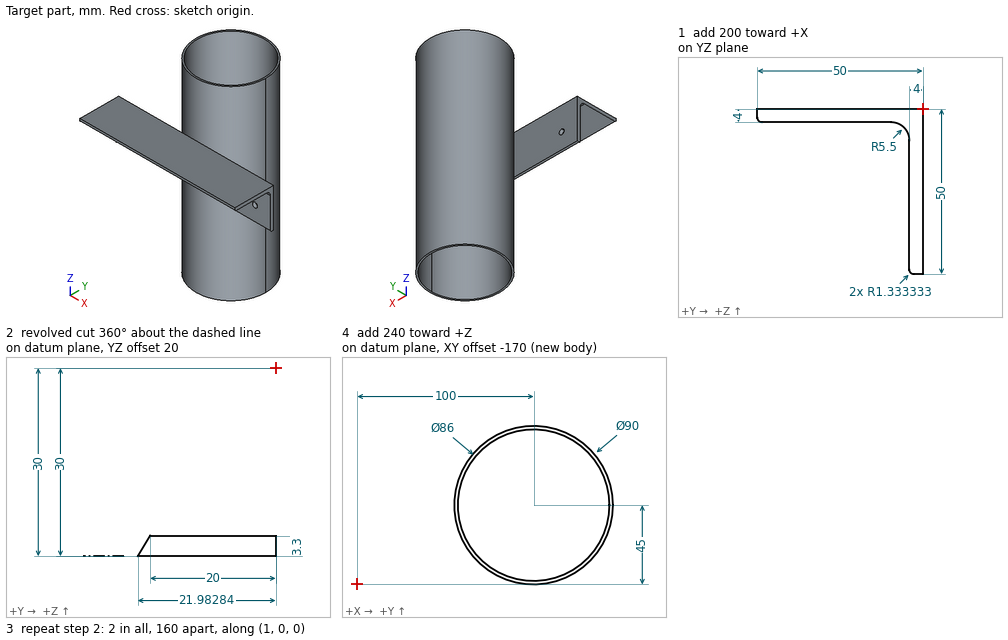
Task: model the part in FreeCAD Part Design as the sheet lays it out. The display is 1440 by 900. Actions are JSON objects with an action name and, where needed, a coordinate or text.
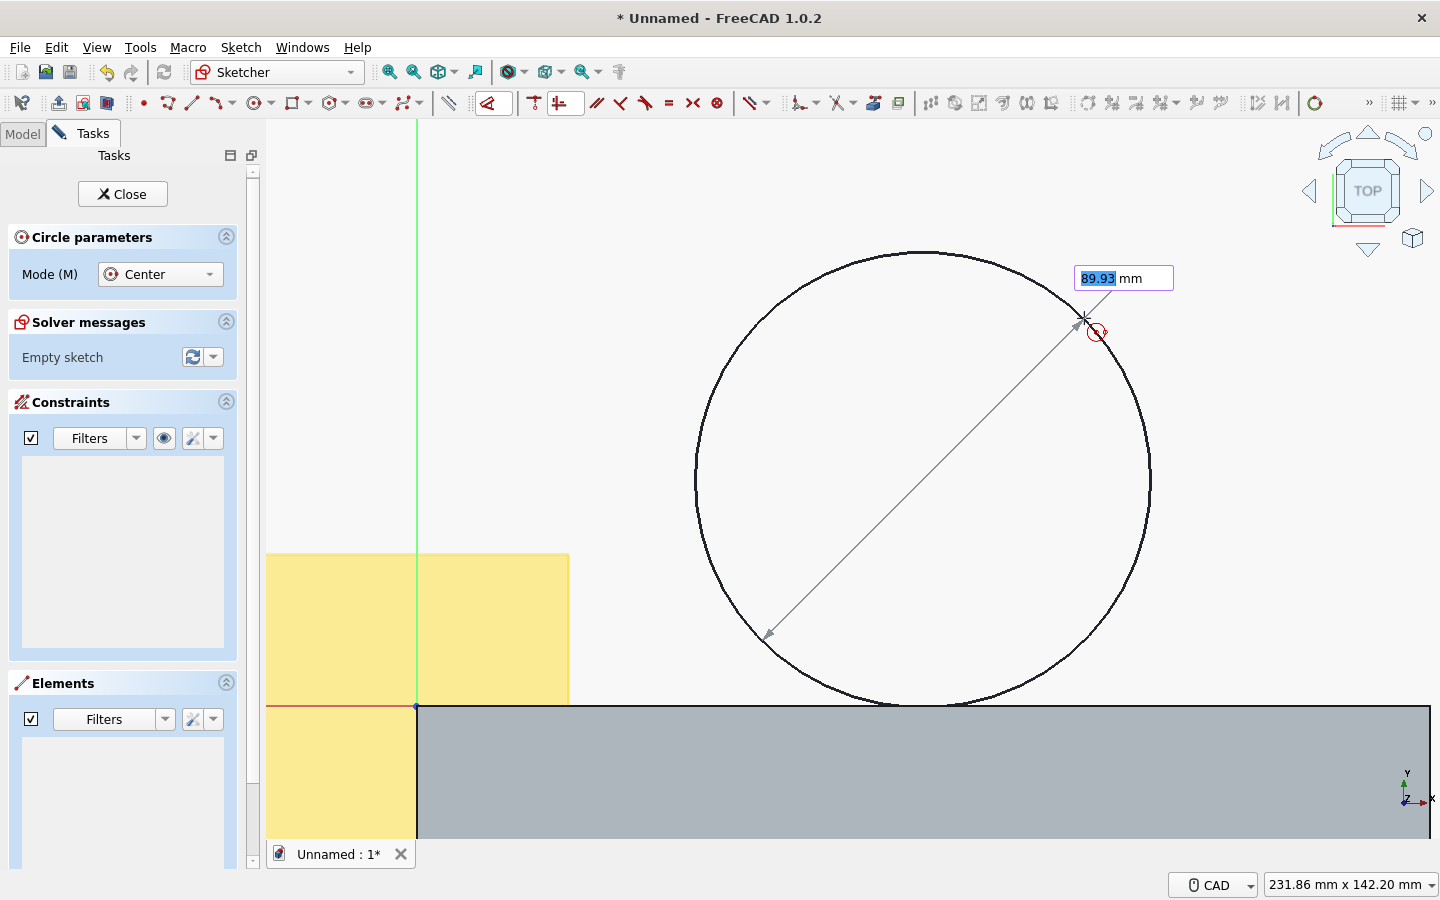
{"action": "type", "text": "90"}
{"action": "key", "text": "Return"}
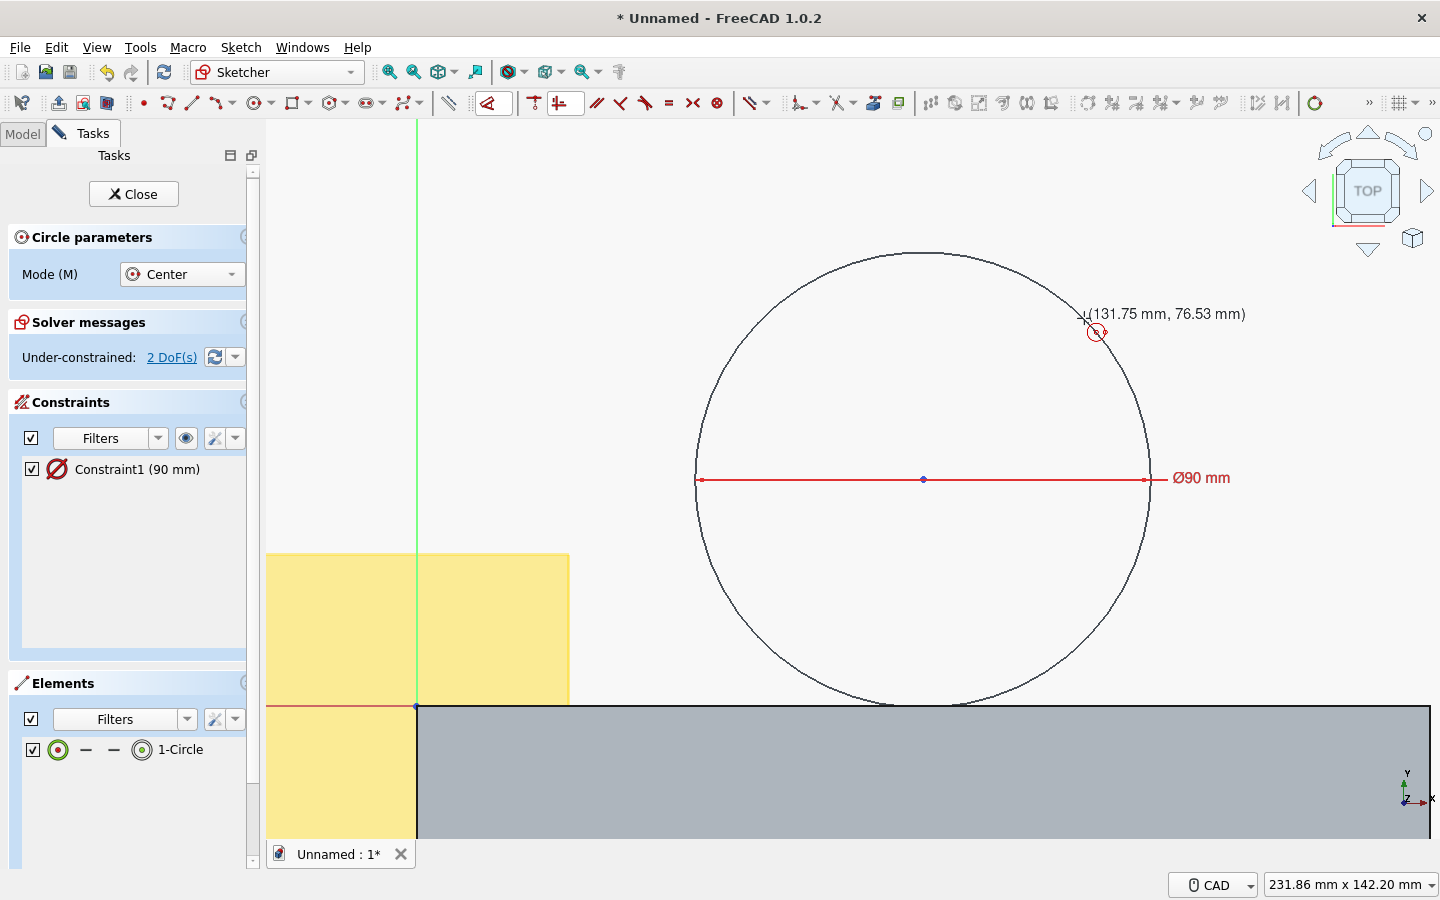
{"action": "left_click", "coordinate": [923, 480]}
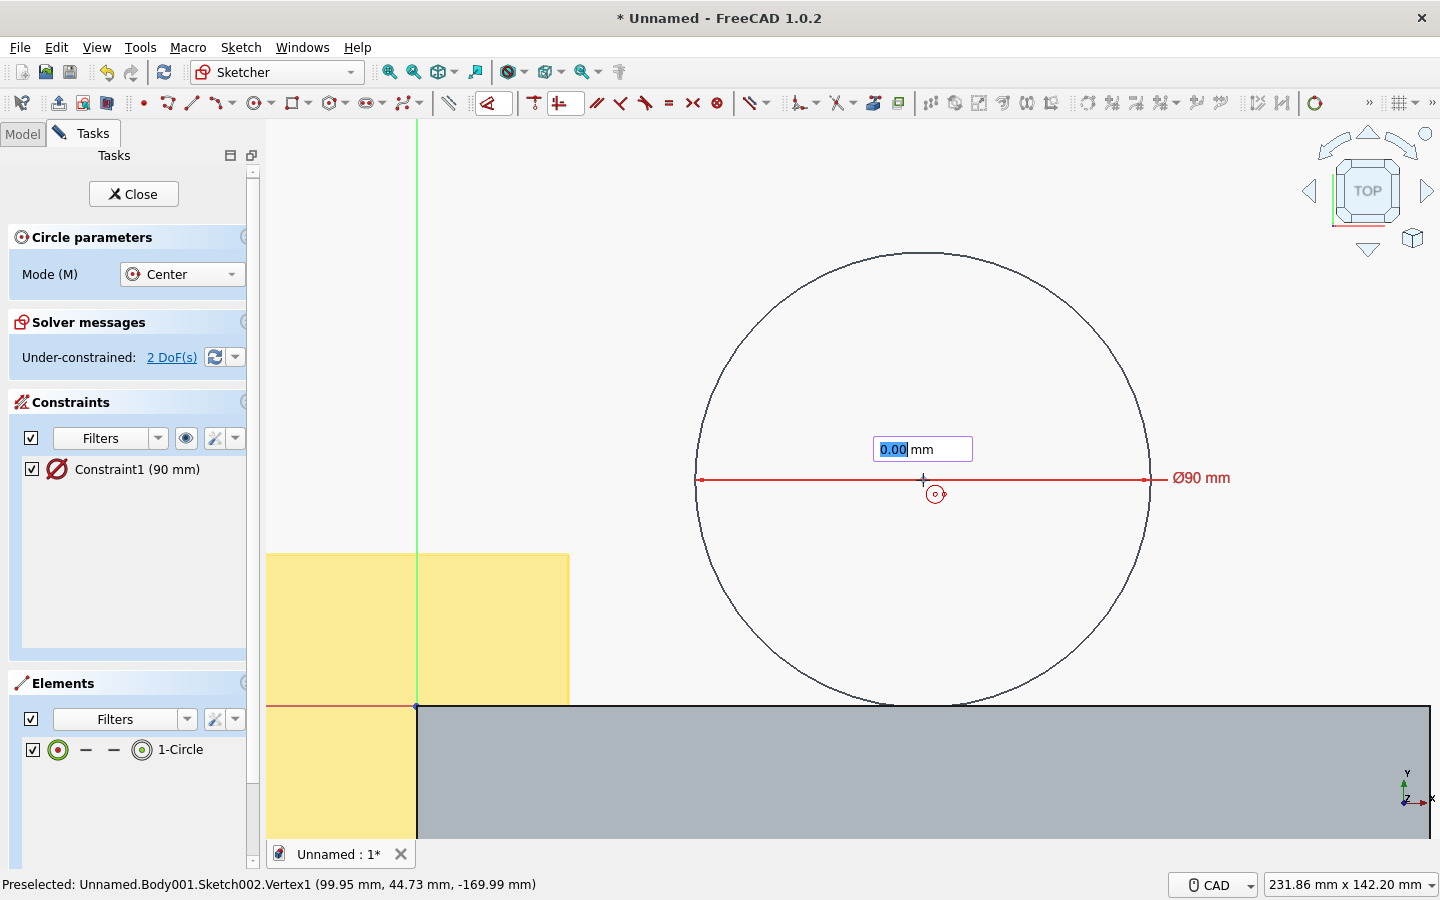
{"action": "scroll", "coordinate": [1077, 325], "scroll_direction": "up", "scroll_amount": 3}
{"action": "mouse_move", "coordinate": [1077, 324]}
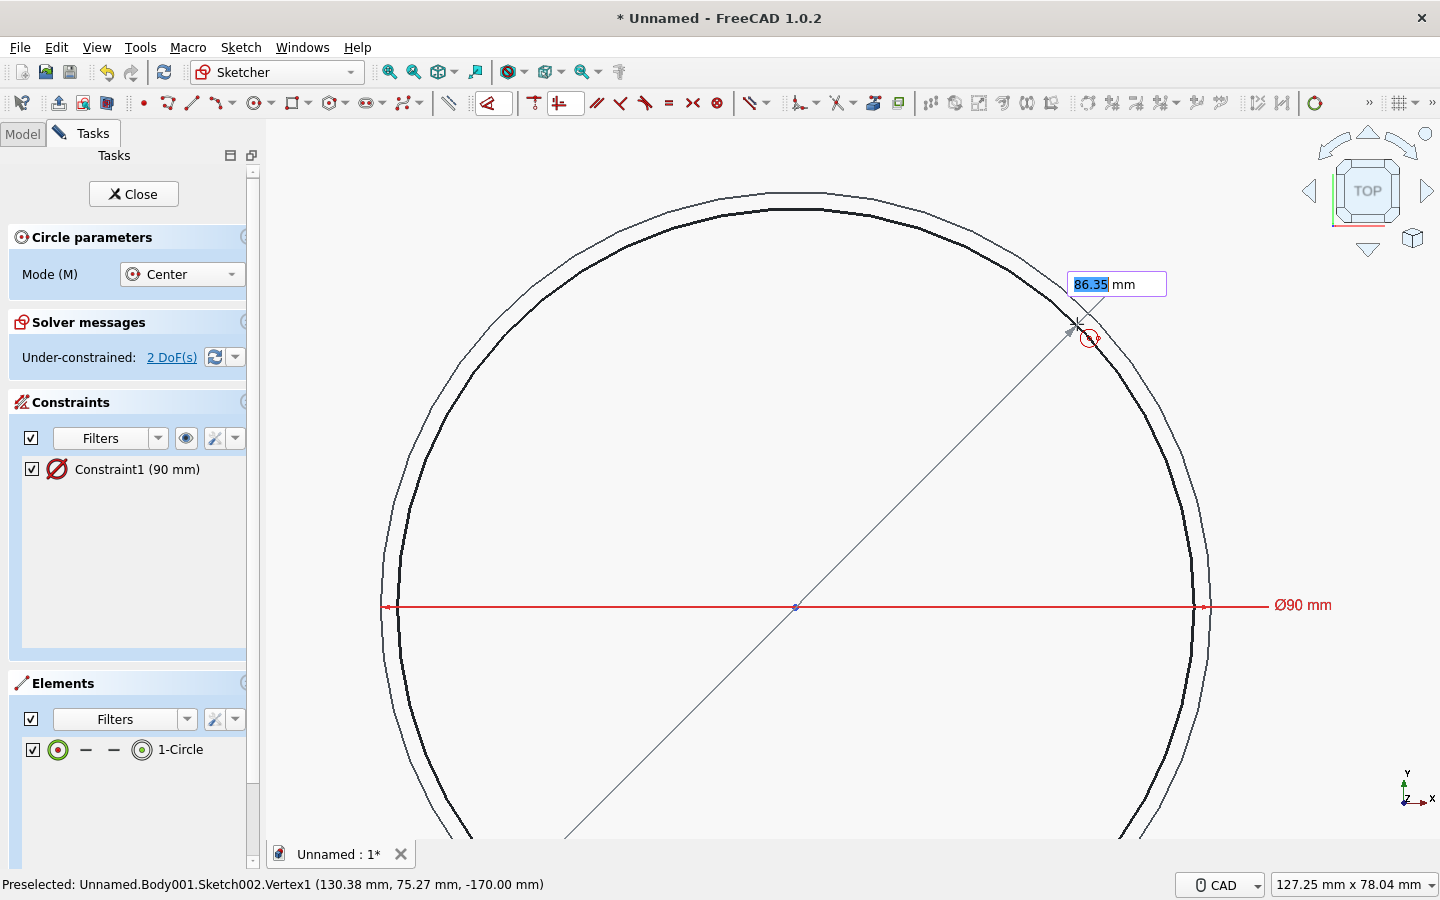
{"action": "type", "text": "86"}
{"action": "key", "text": "Return"}
{"action": "key", "text": "Escape"}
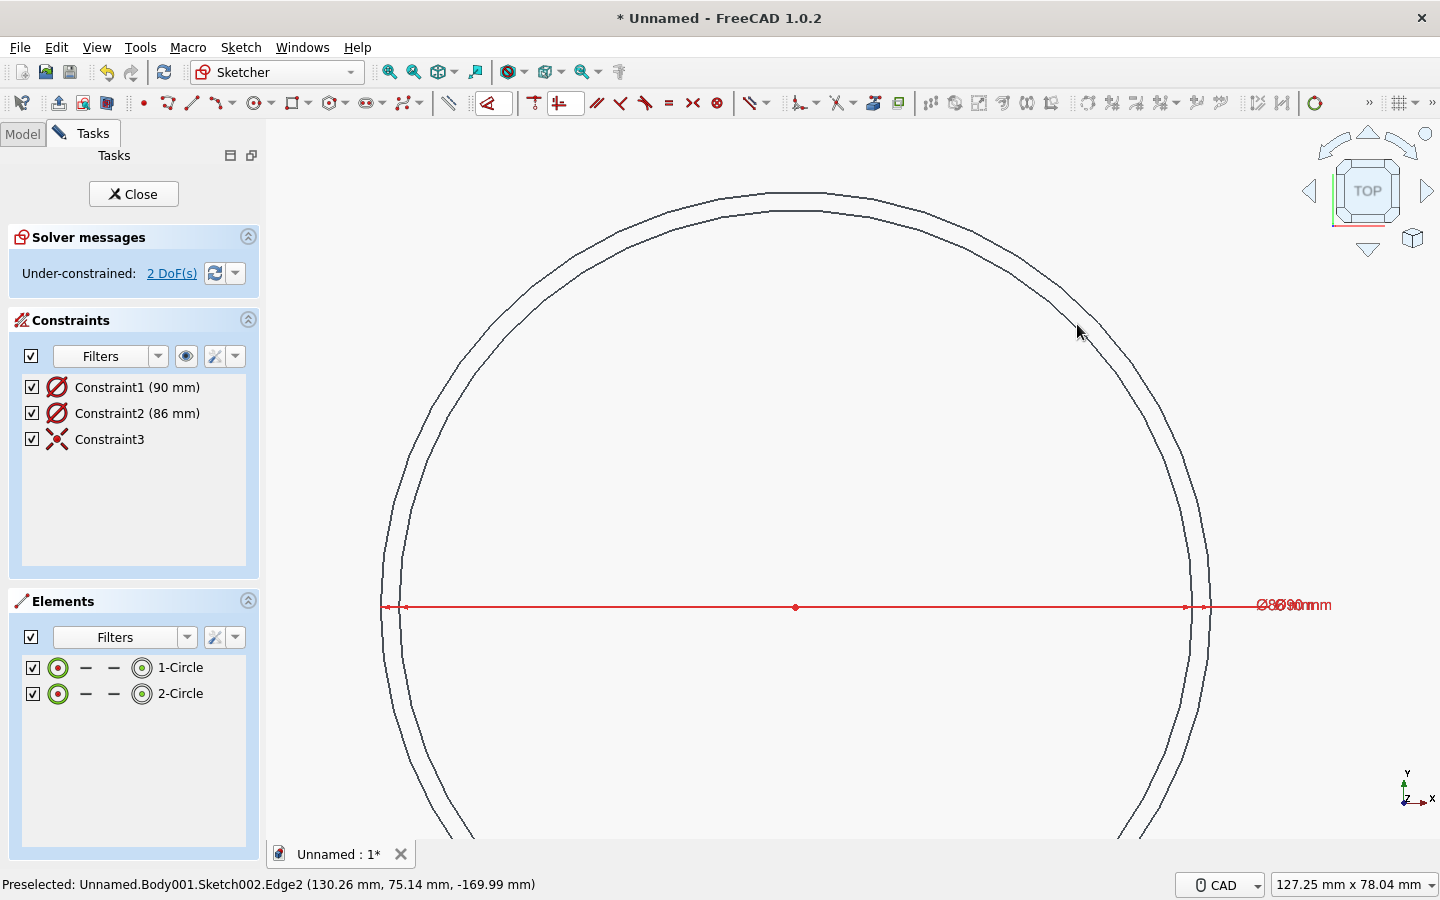
{"action": "left_click", "coordinate": [796, 607]}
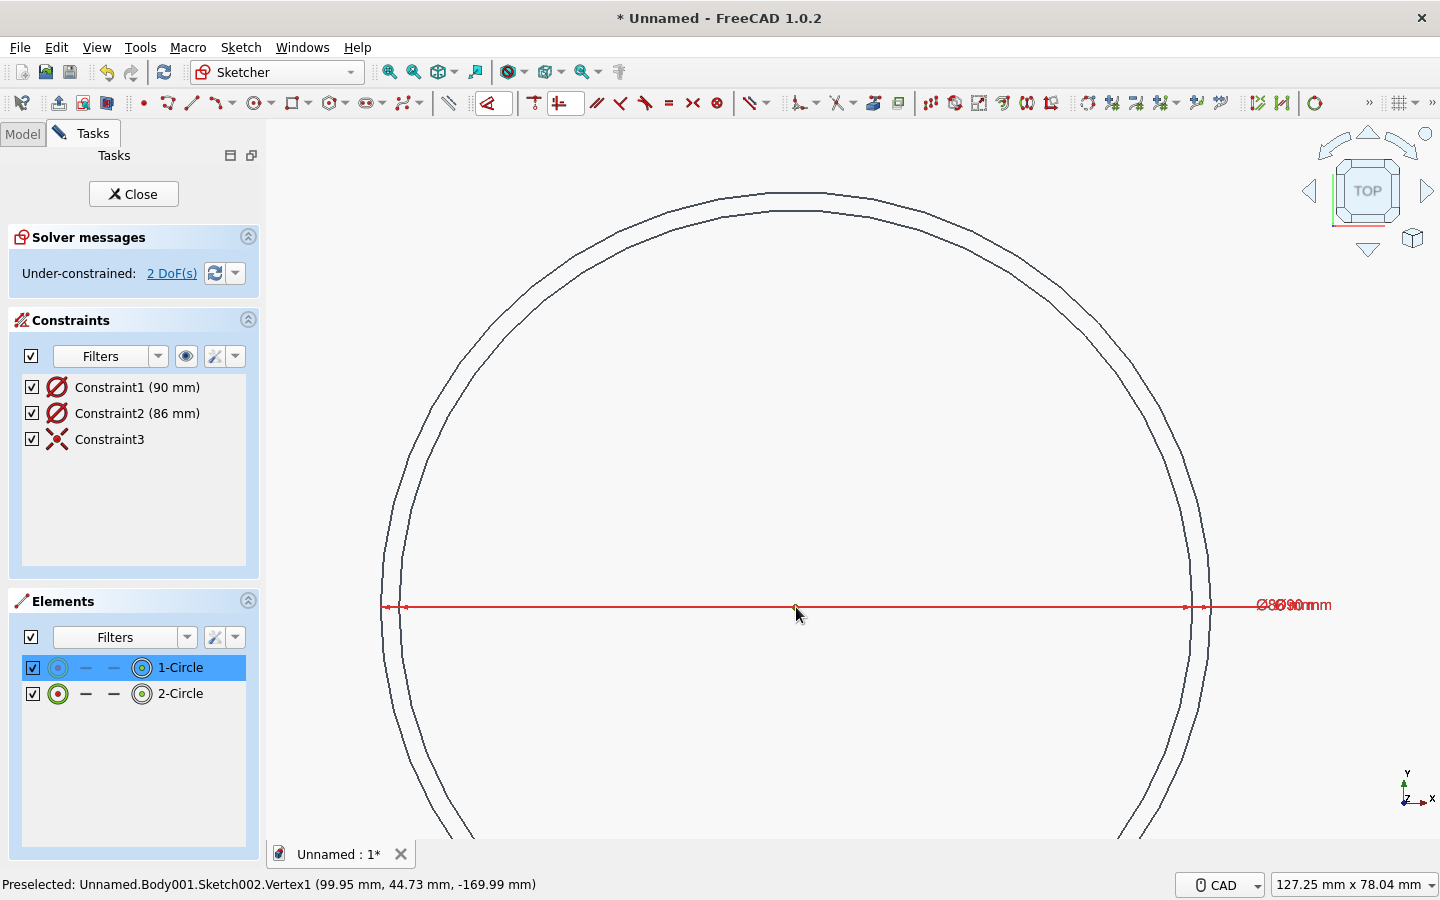
{"action": "key", "text": "i"}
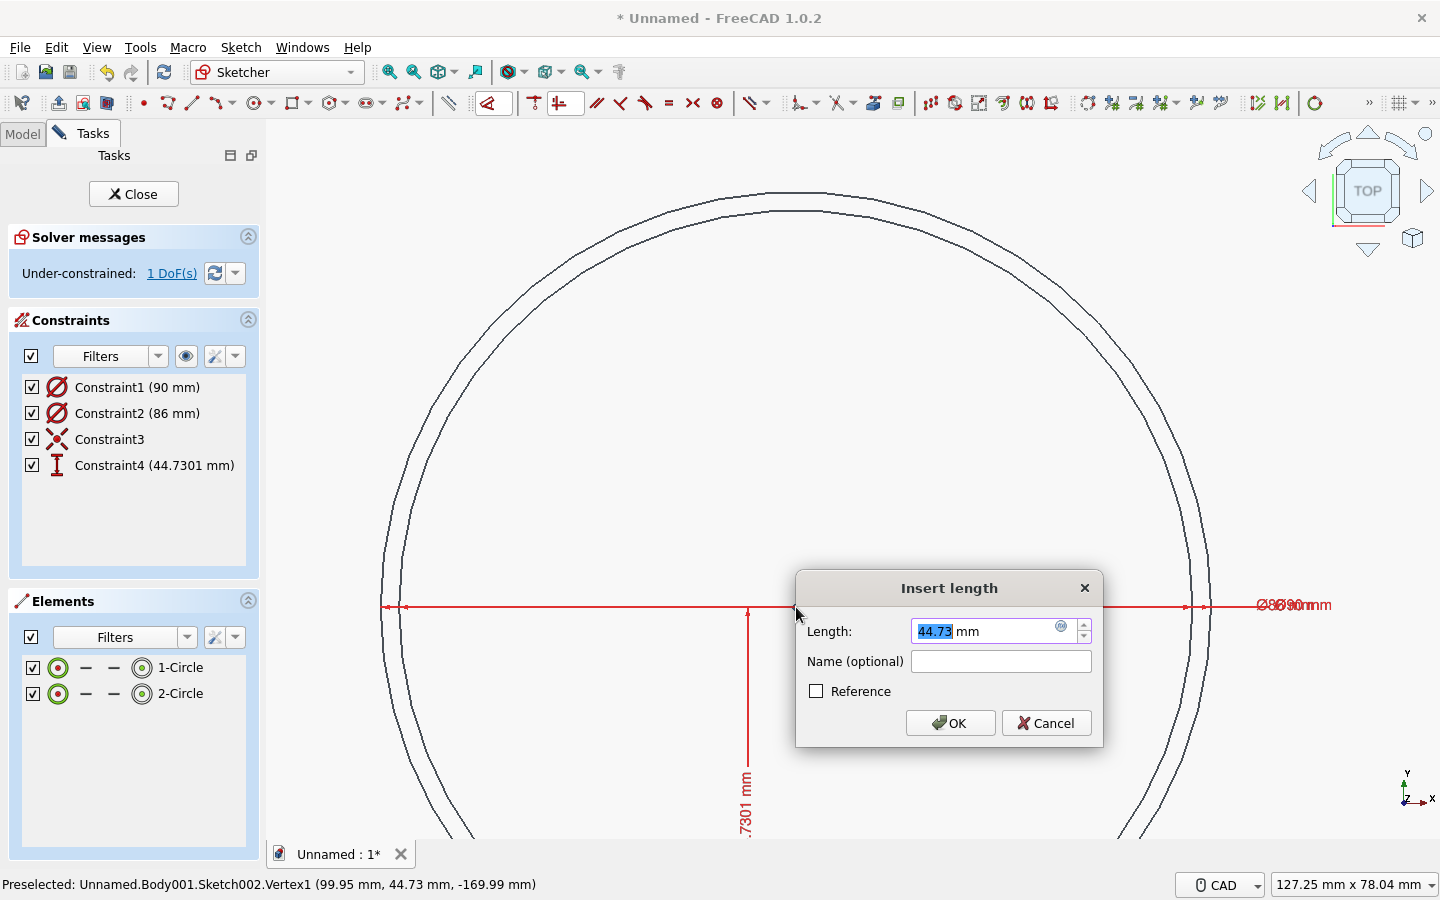
{"action": "type", "text": "45"}
{"action": "key", "text": "Return"}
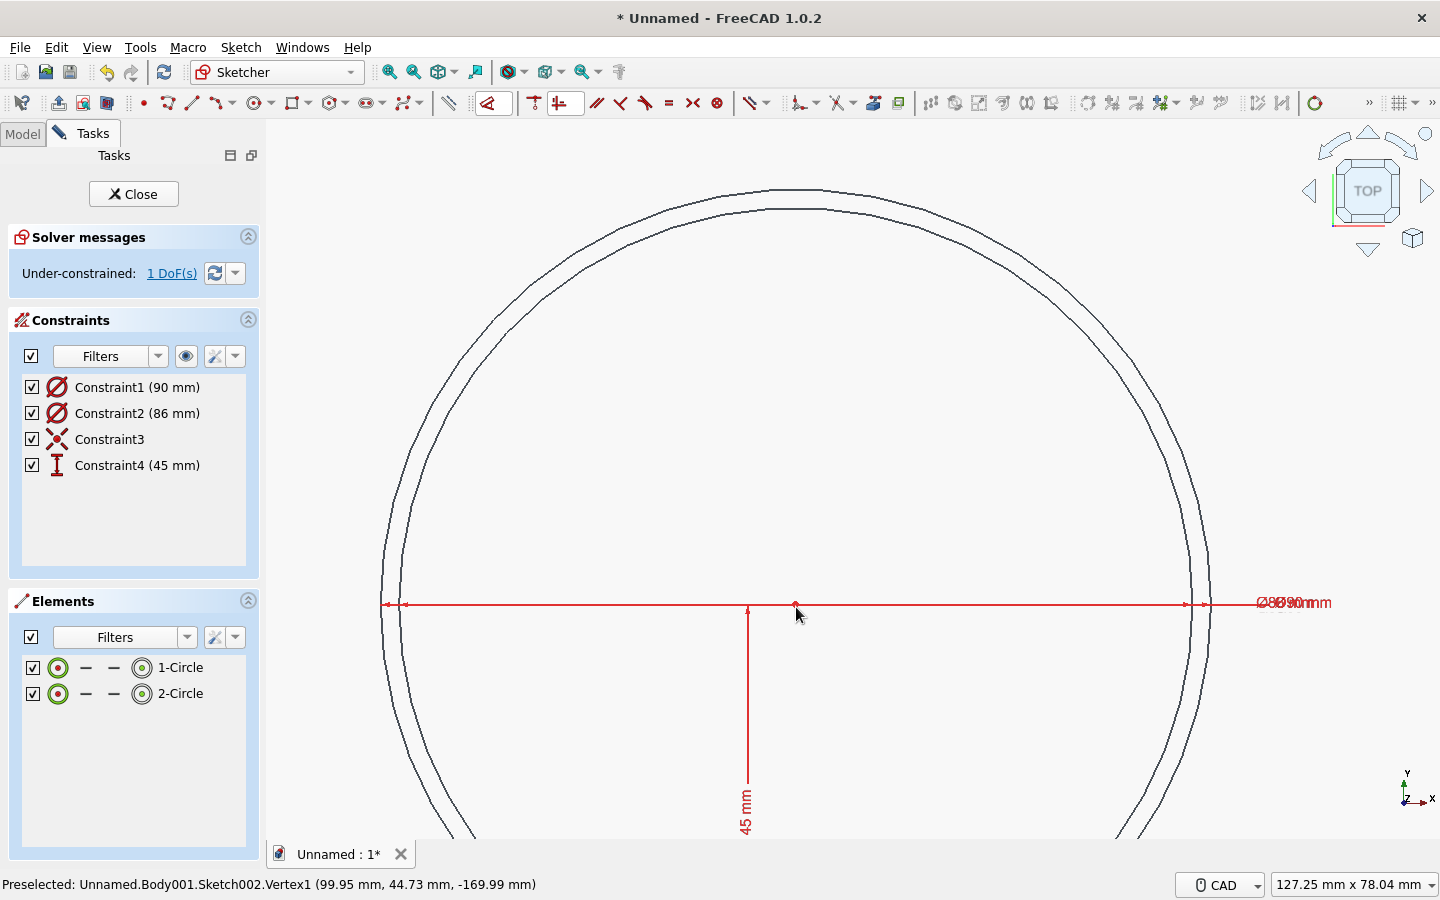
{"action": "left_click", "coordinate": [796, 605]}